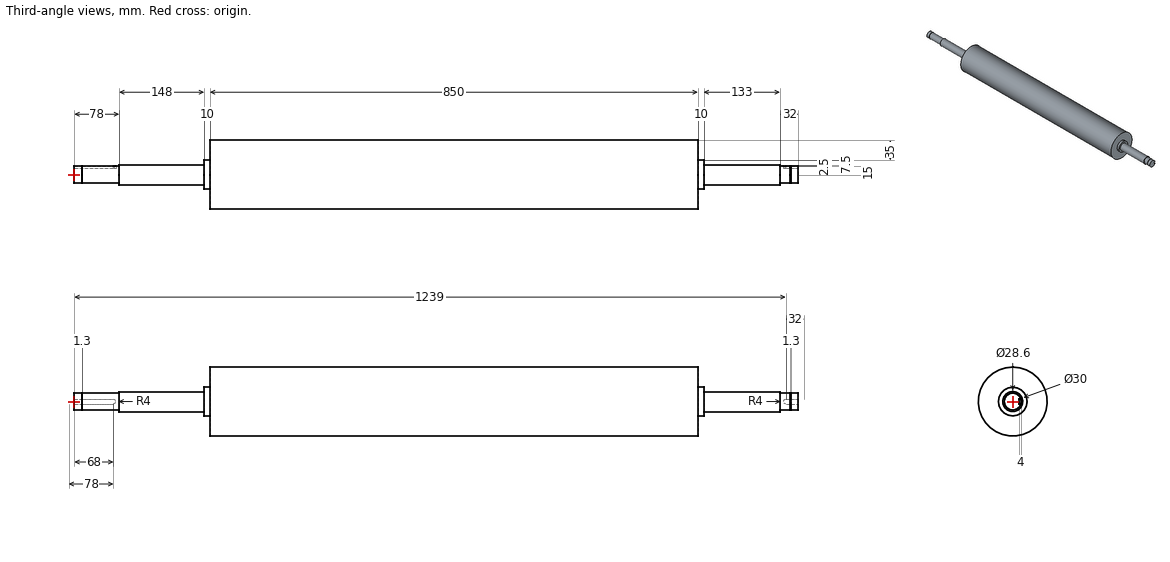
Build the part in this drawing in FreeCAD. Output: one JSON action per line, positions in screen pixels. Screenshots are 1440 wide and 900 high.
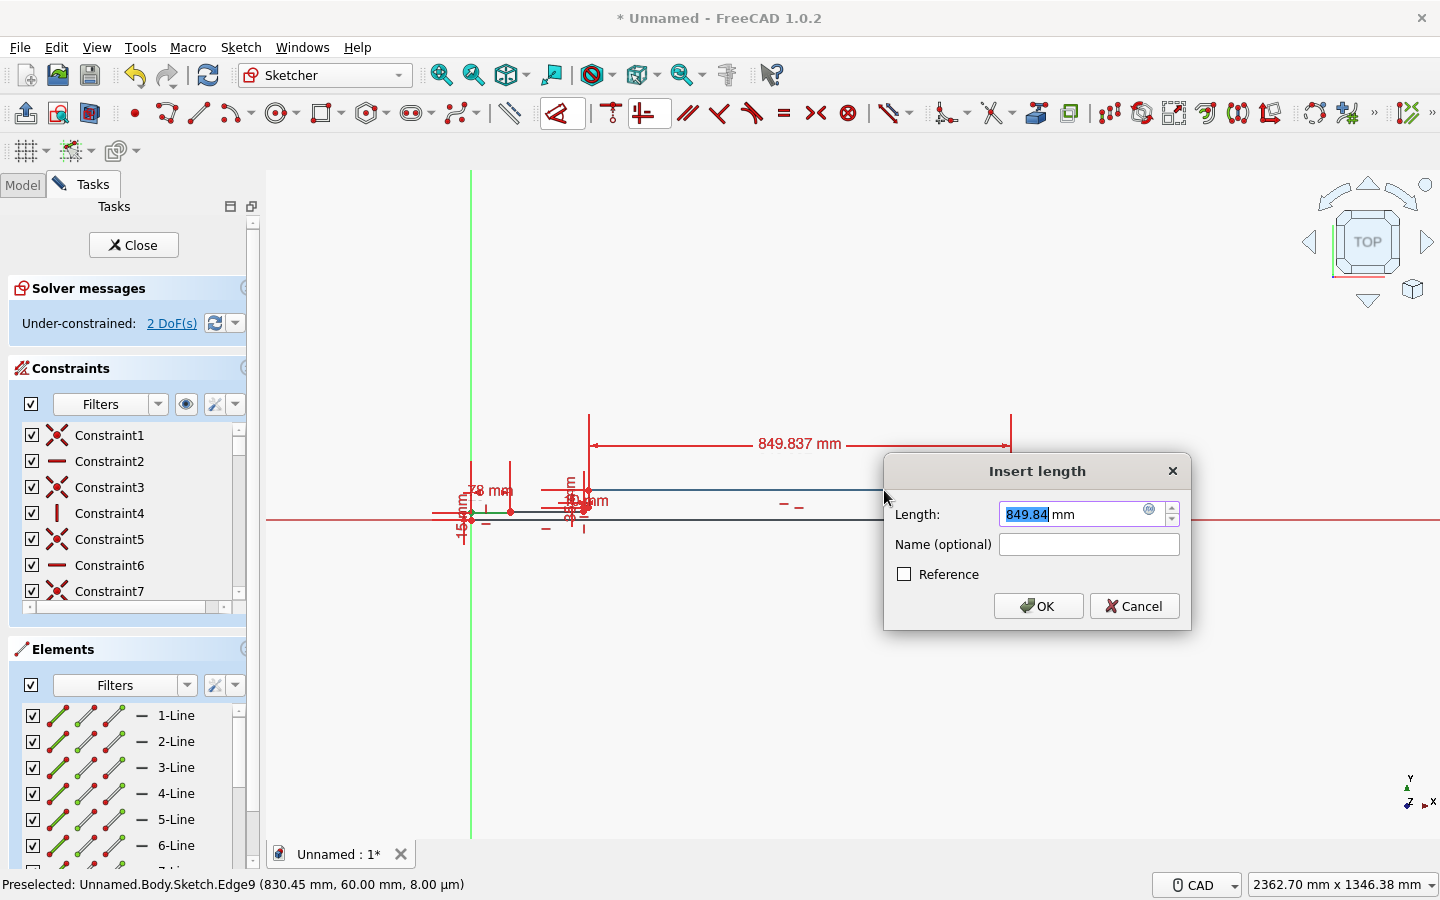
{"action": "type", "text": "850"}
{"action": "key", "text": "Return"}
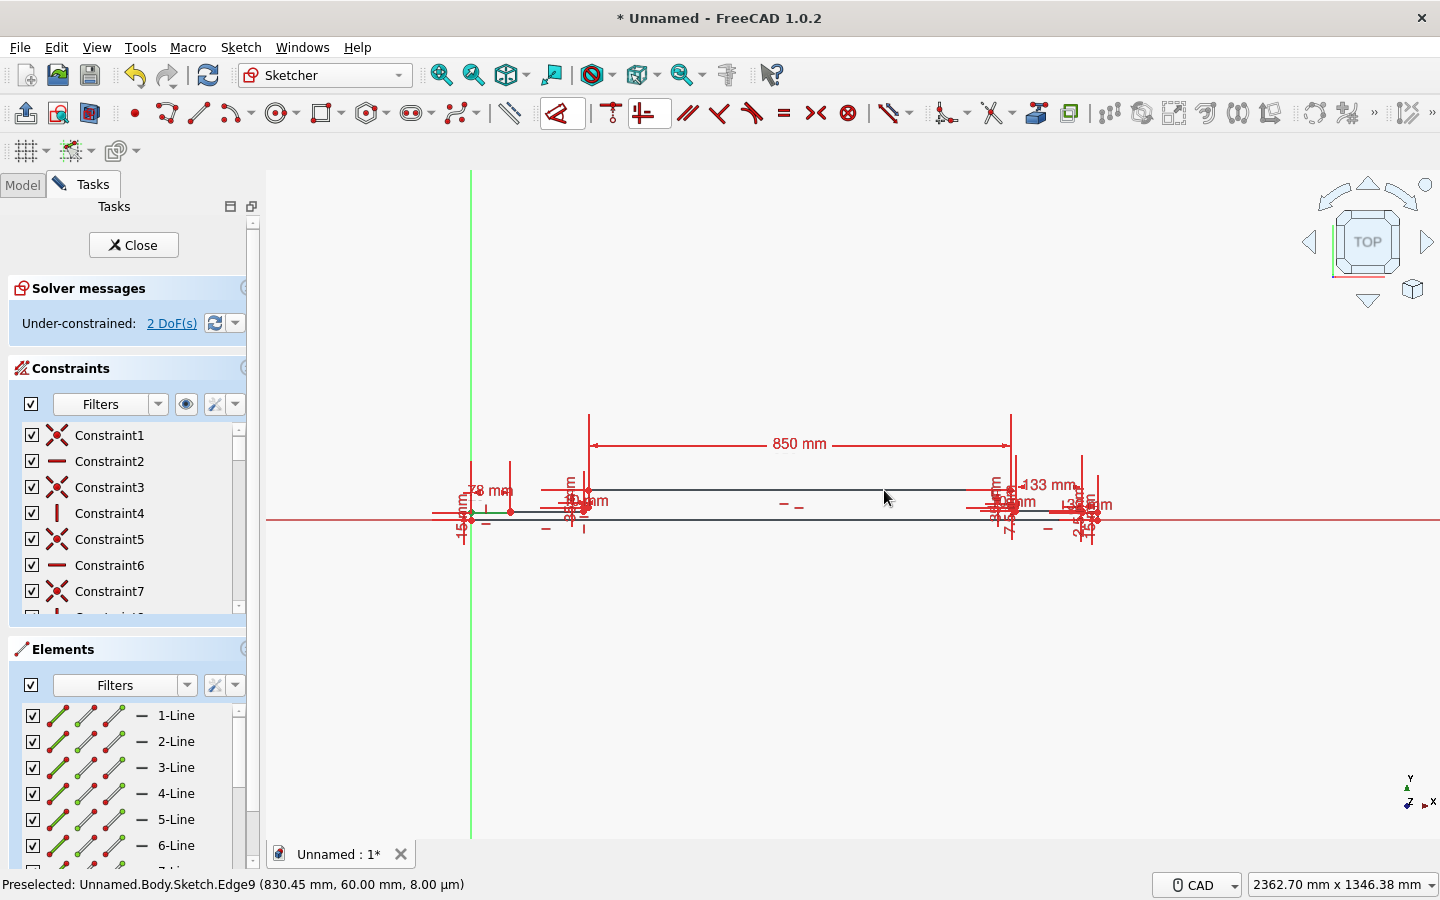
{"action": "scroll", "coordinate": [584, 510], "scroll_direction": "up", "scroll_amount": 12}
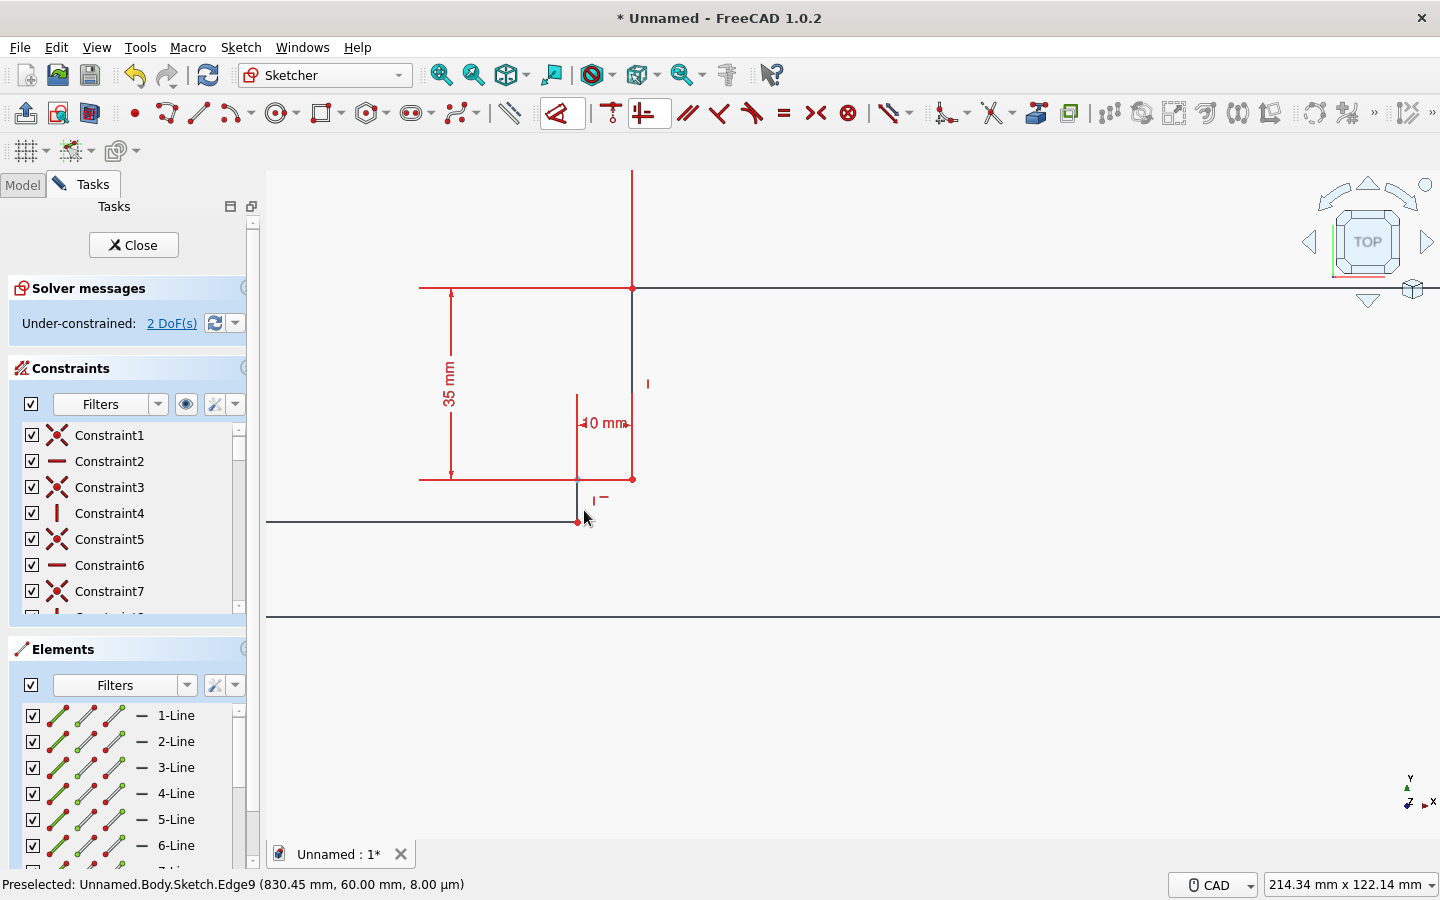
{"action": "left_click", "coordinate": [577, 501]}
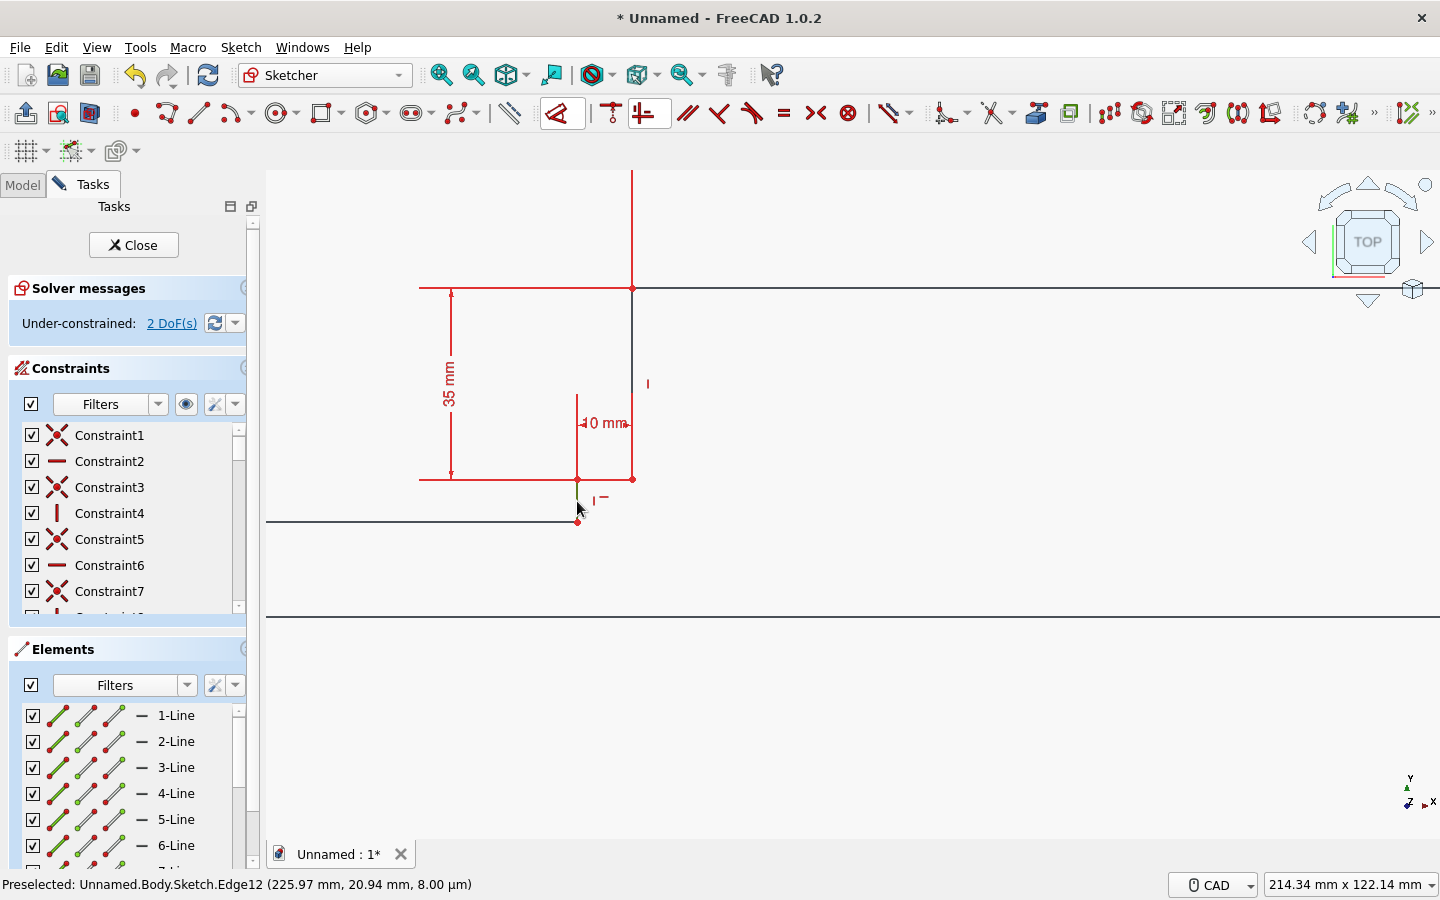
{"action": "key", "text": "i"}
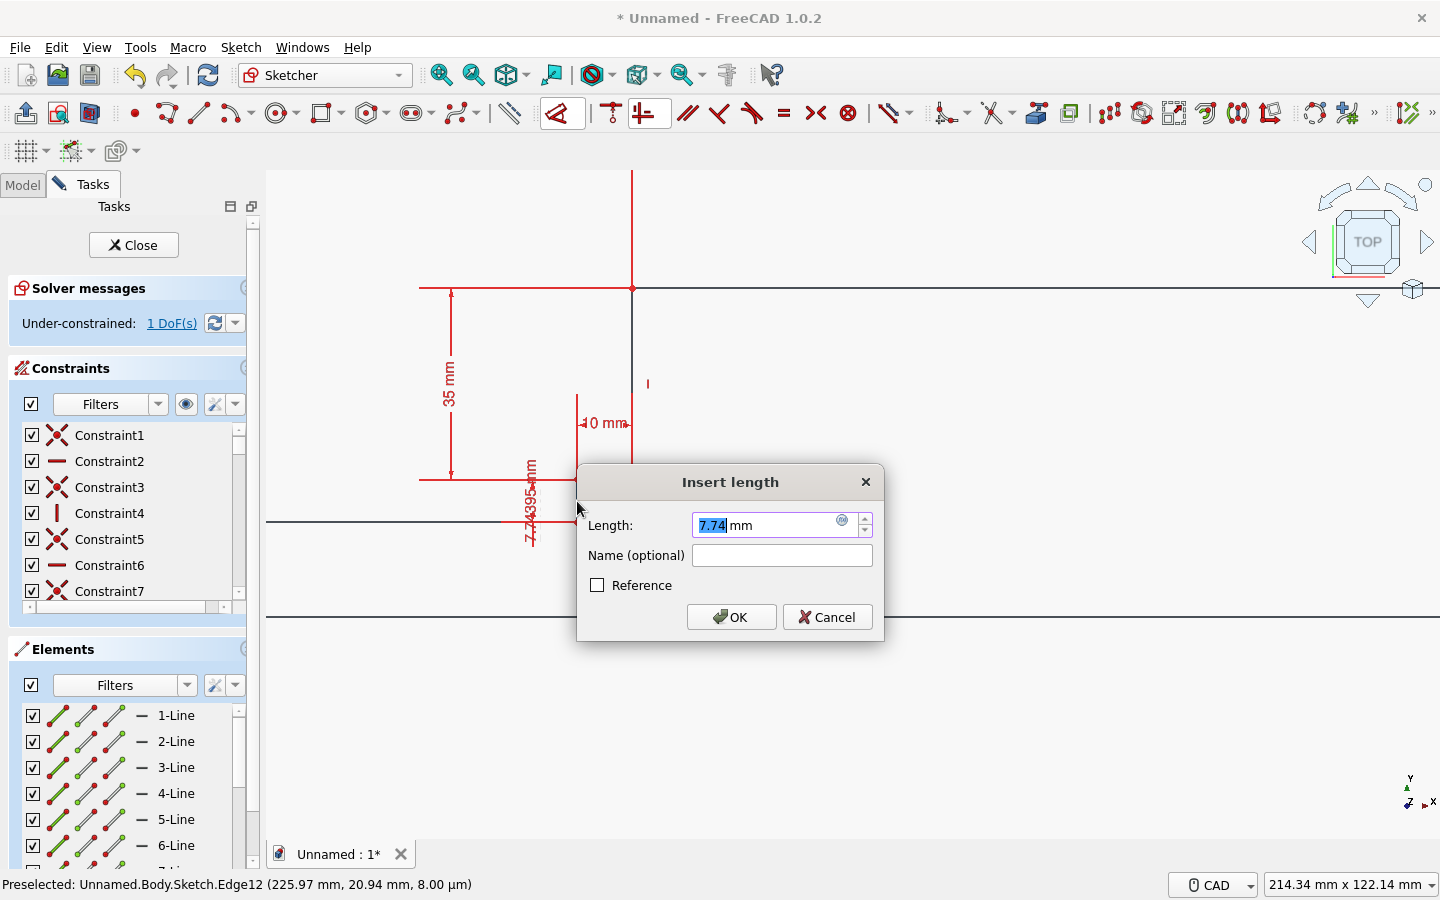
{"action": "type", "text": "7.5"}
{"action": "key", "text": "Return"}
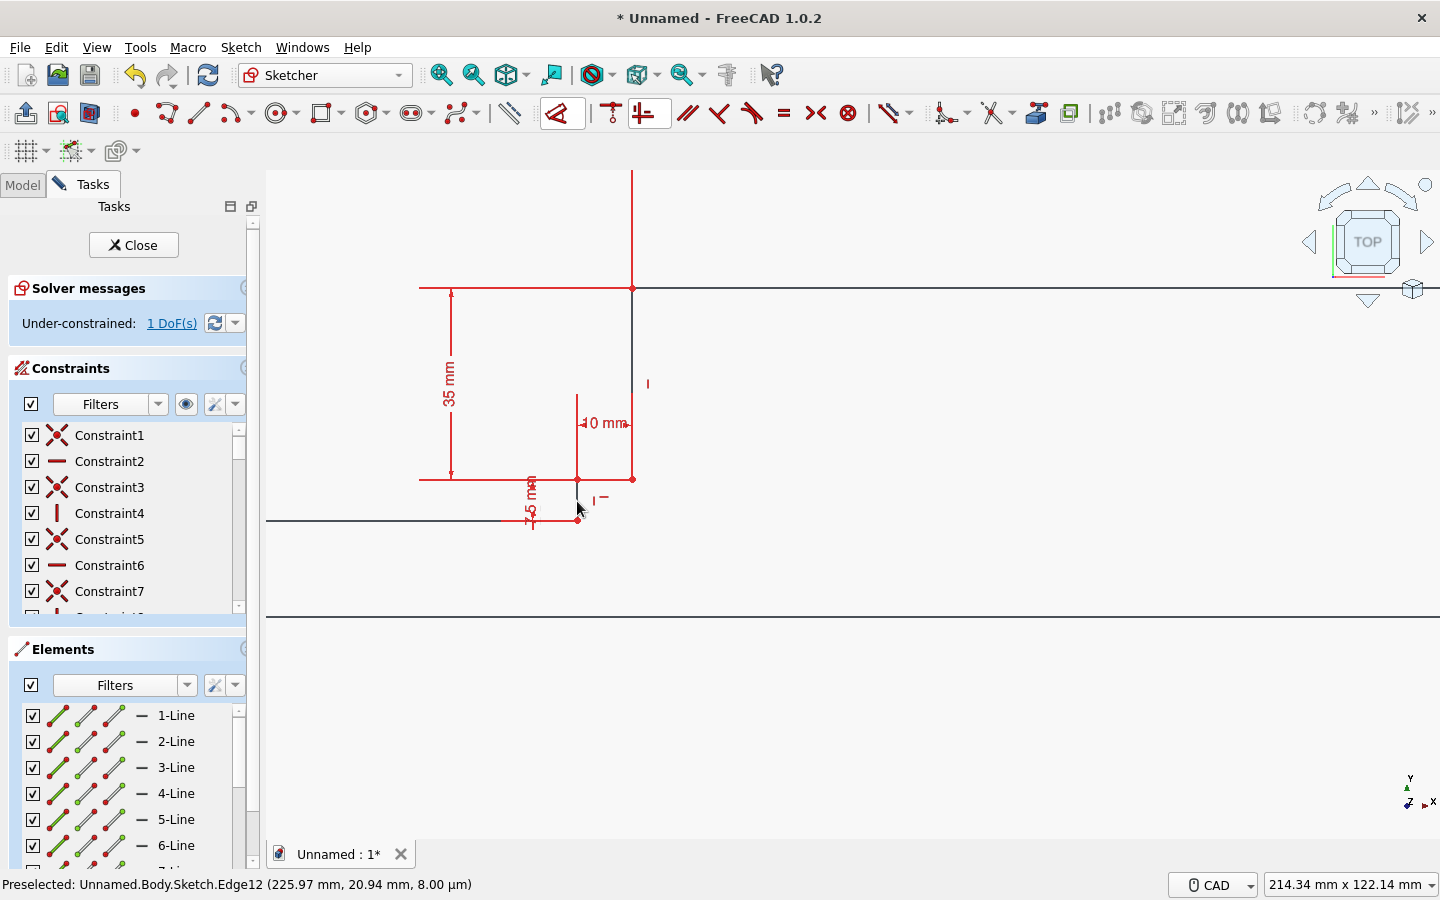
{"action": "scroll", "coordinate": [584, 510], "scroll_direction": "down", "scroll_amount": 12}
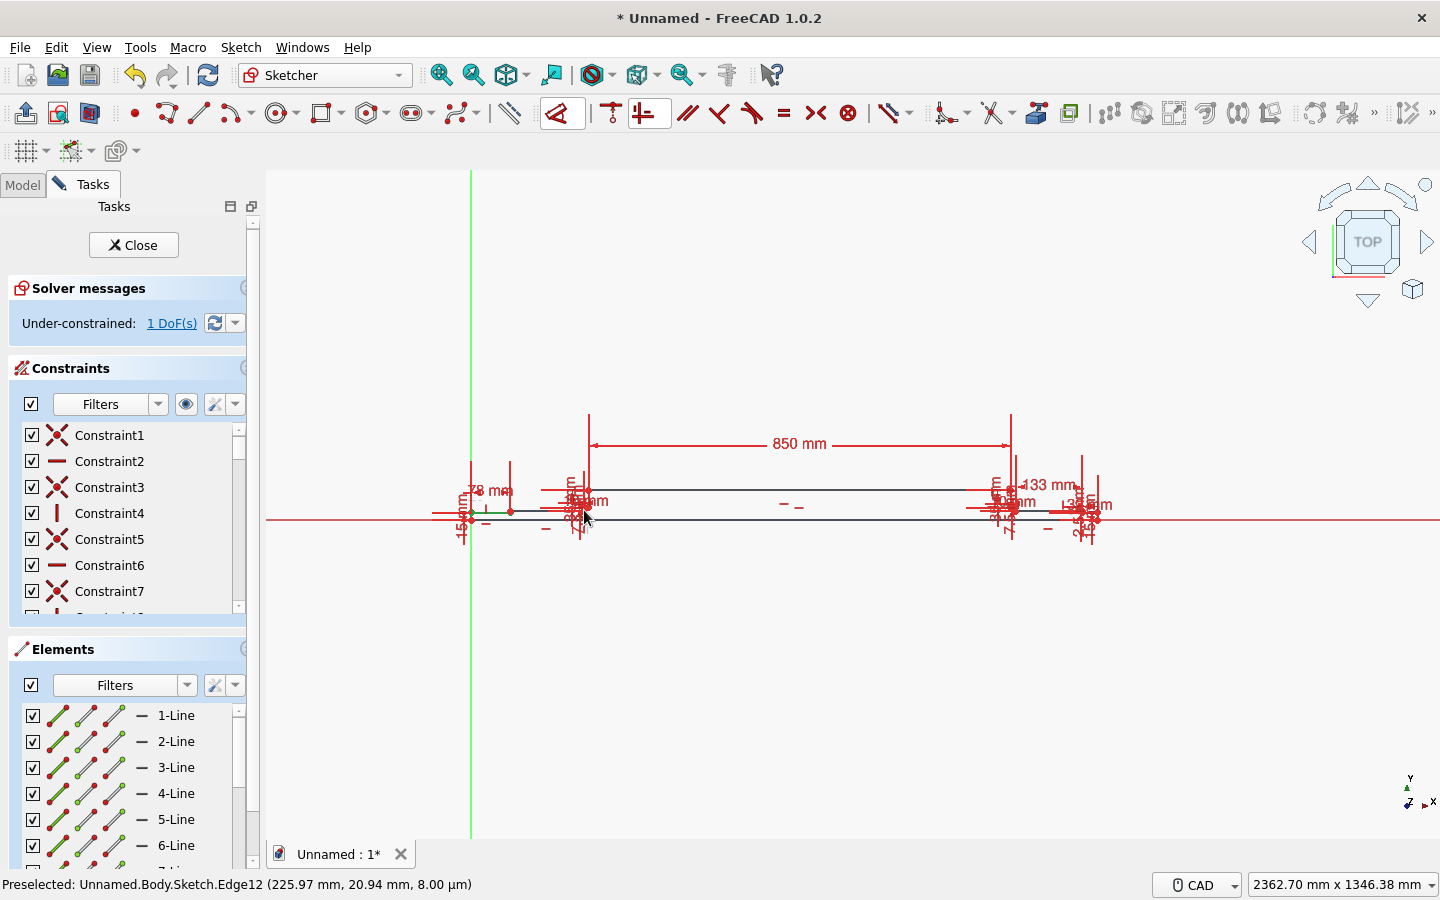
{"action": "scroll", "coordinate": [562, 511], "scroll_direction": "up", "scroll_amount": 3}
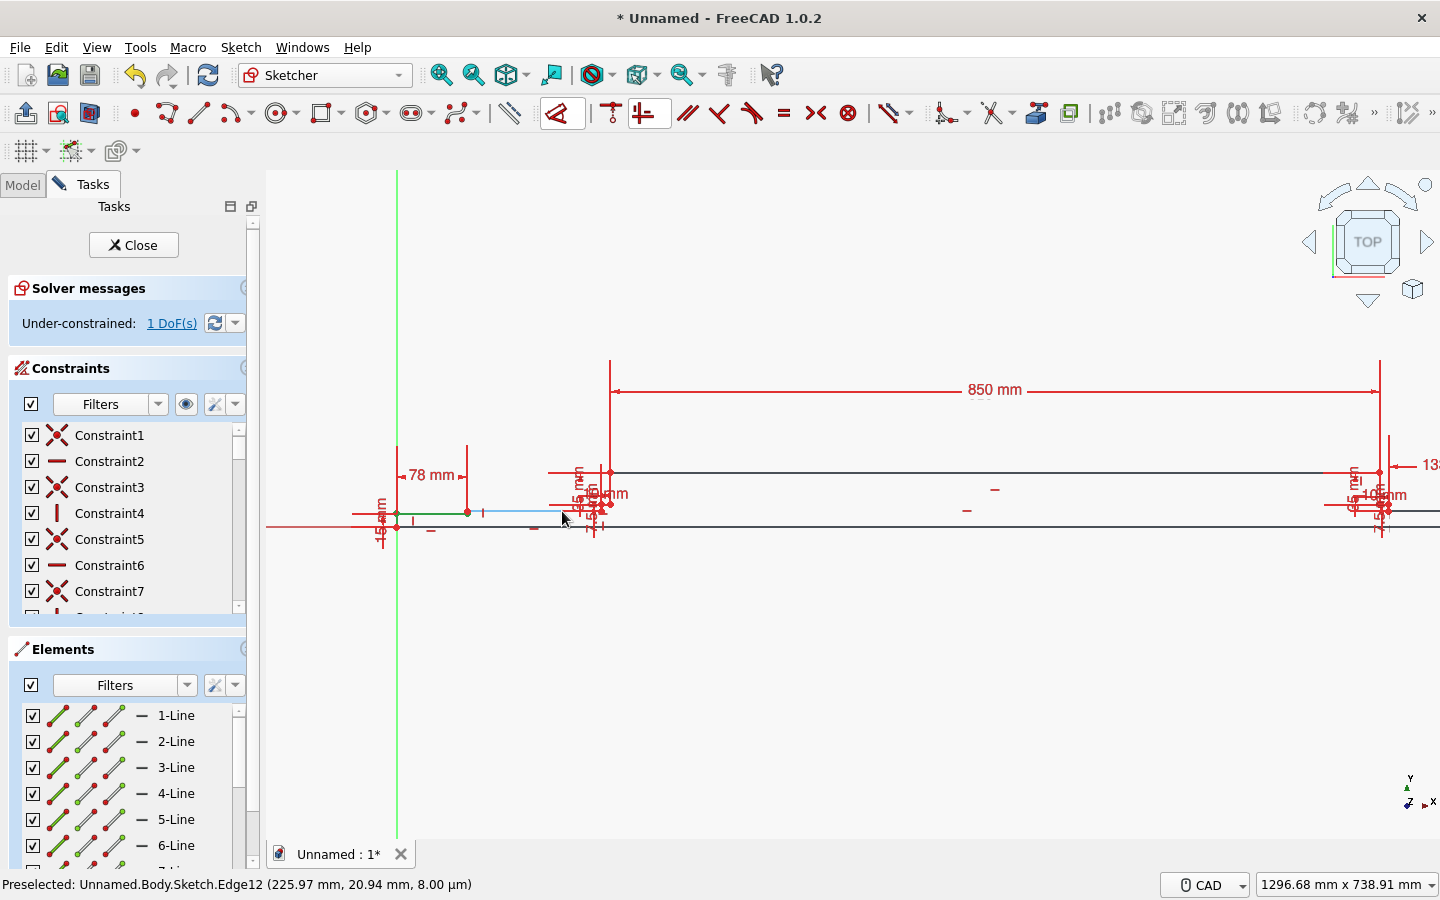
{"action": "left_click", "coordinate": [561, 511]}